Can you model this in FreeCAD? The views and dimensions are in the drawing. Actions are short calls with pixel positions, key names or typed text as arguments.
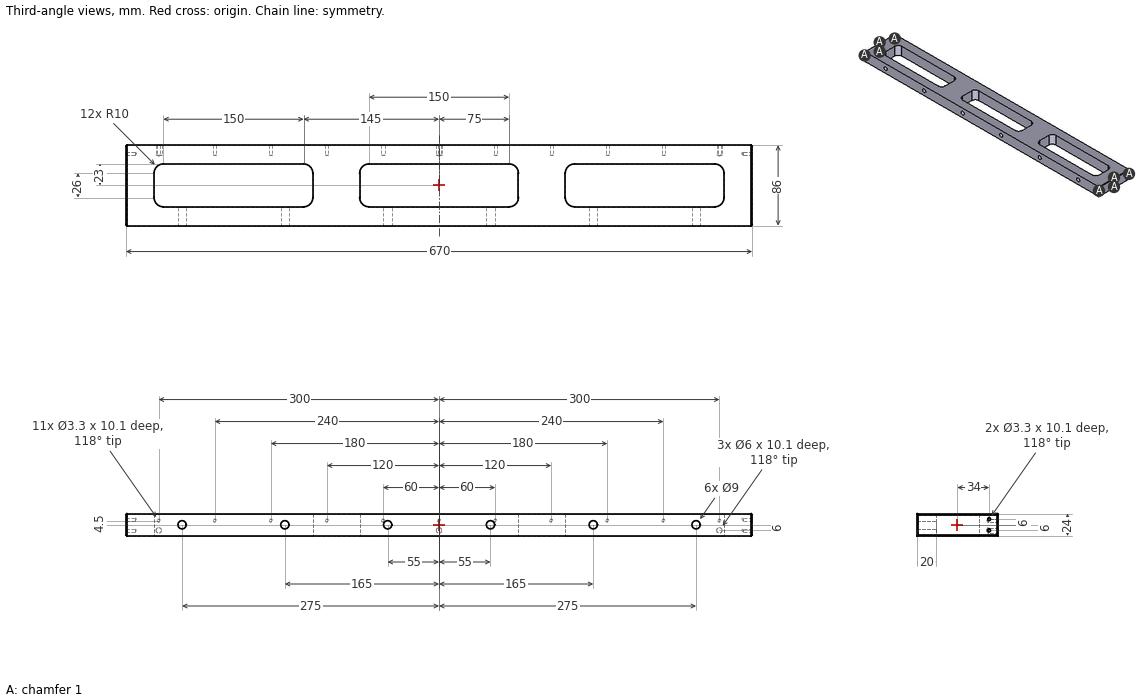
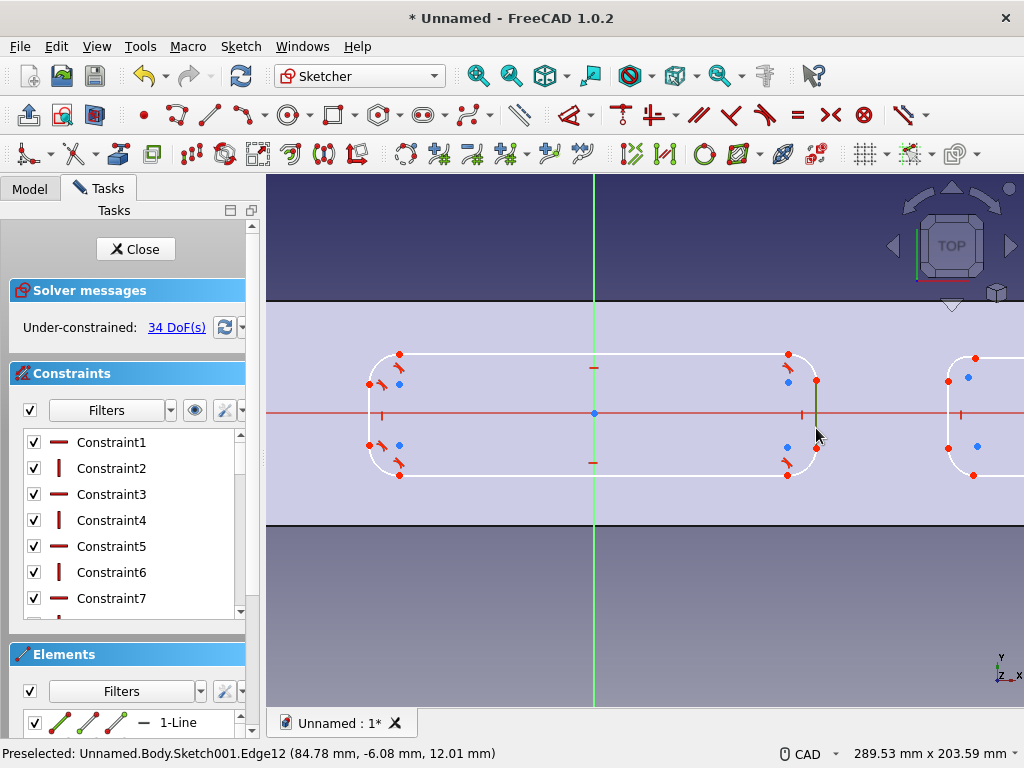
click(800, 473)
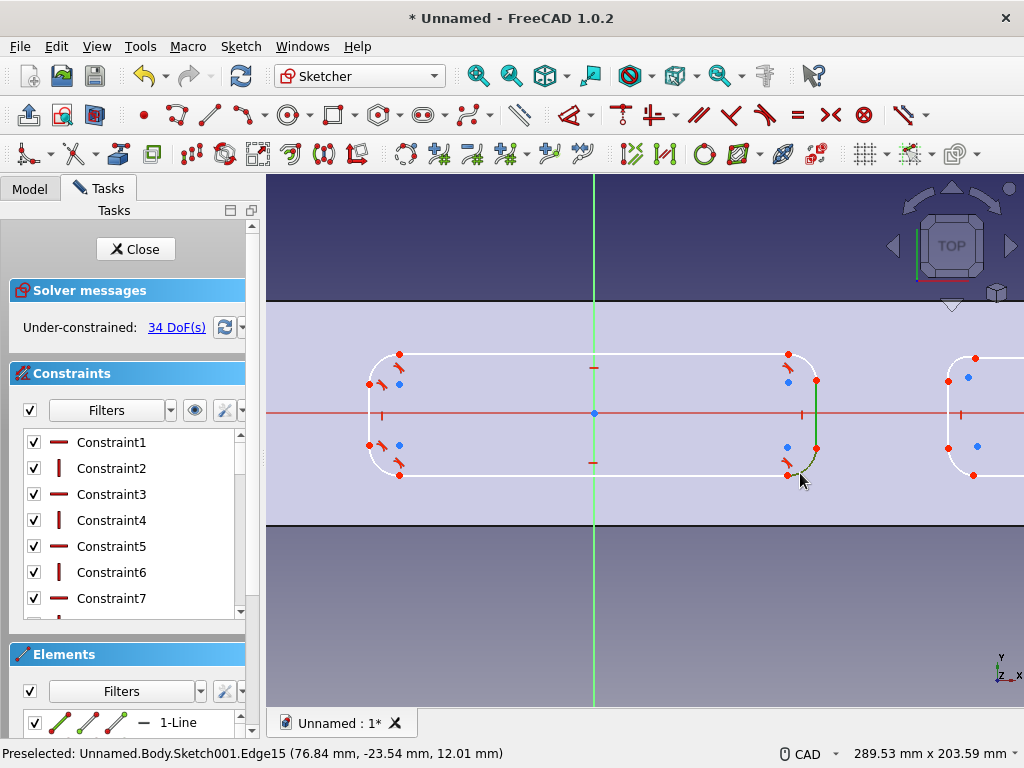
key(t)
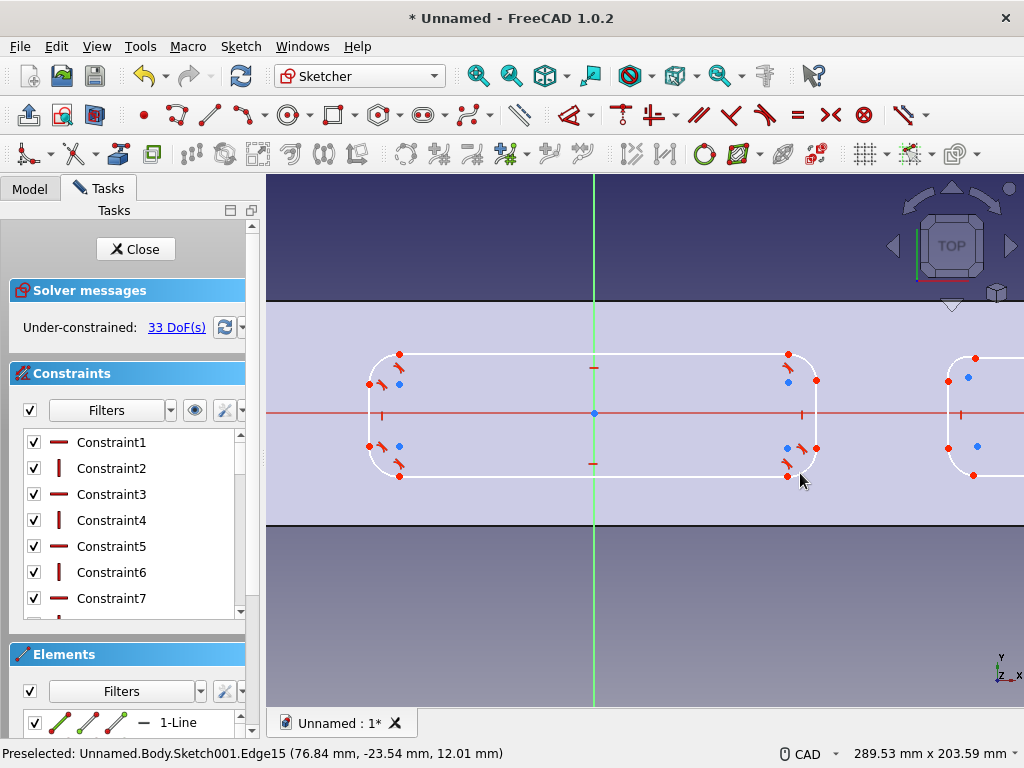
click(816, 428)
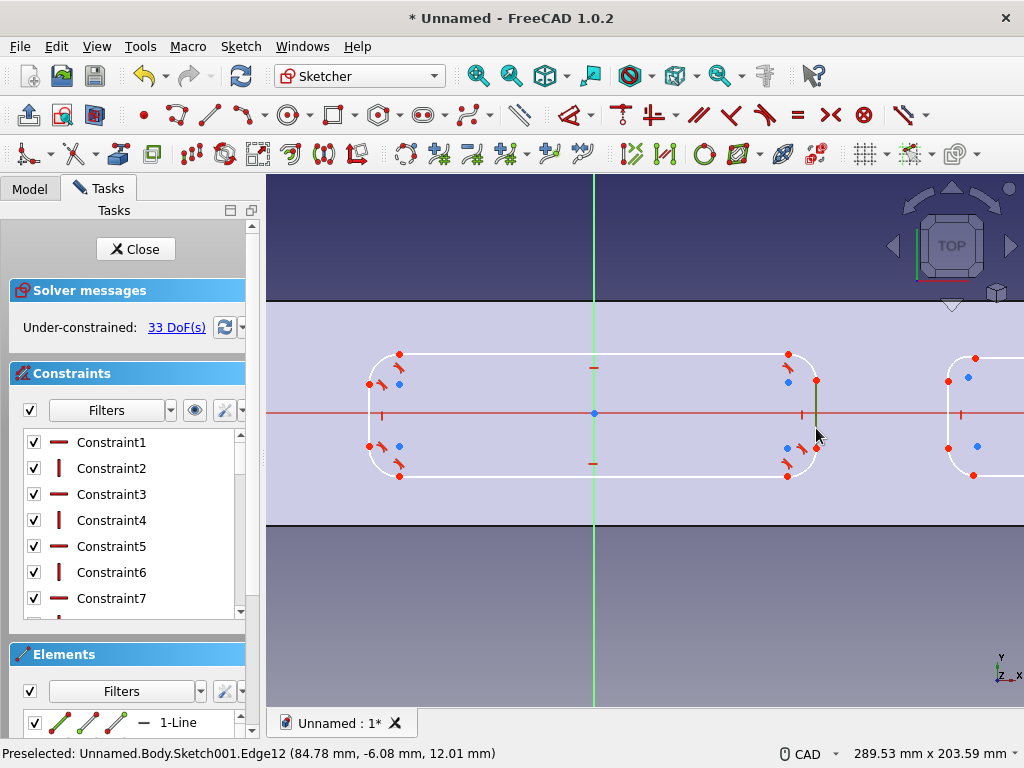
click(813, 369)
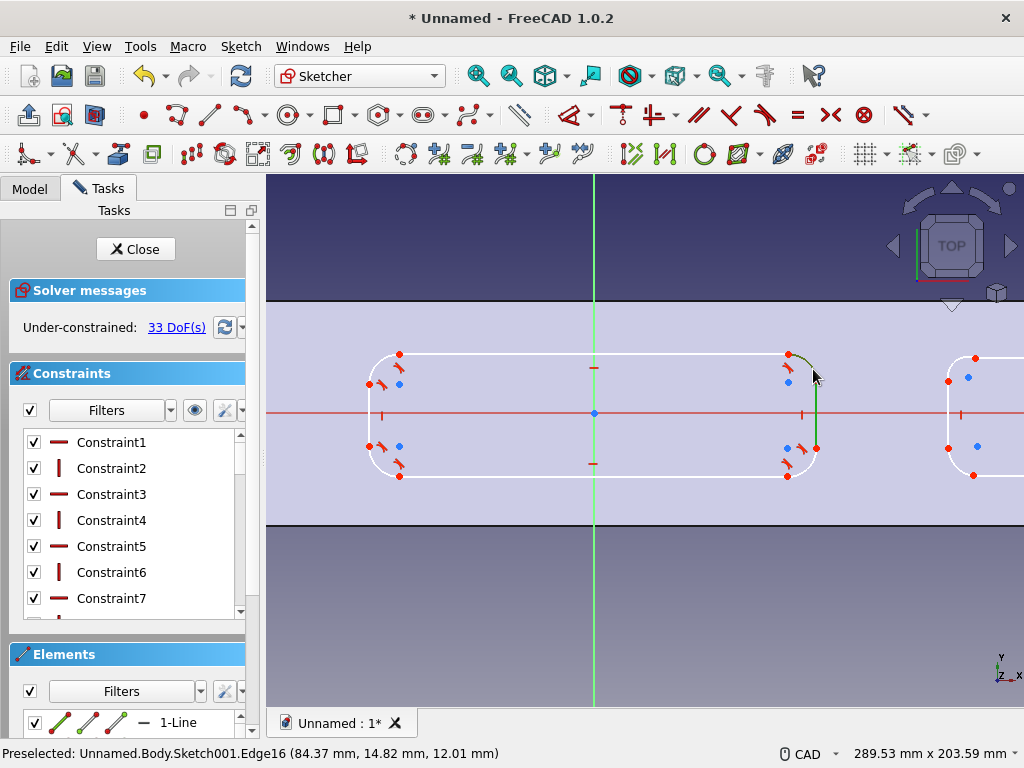
click(765, 116)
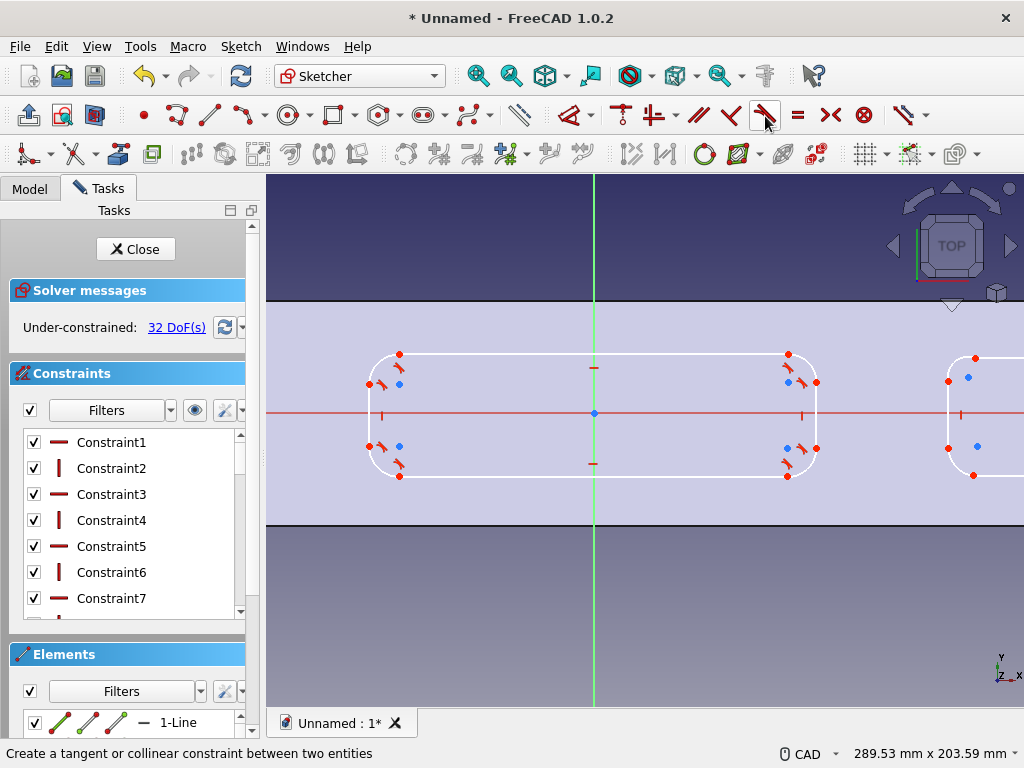
scroll(571, 449, down, 7)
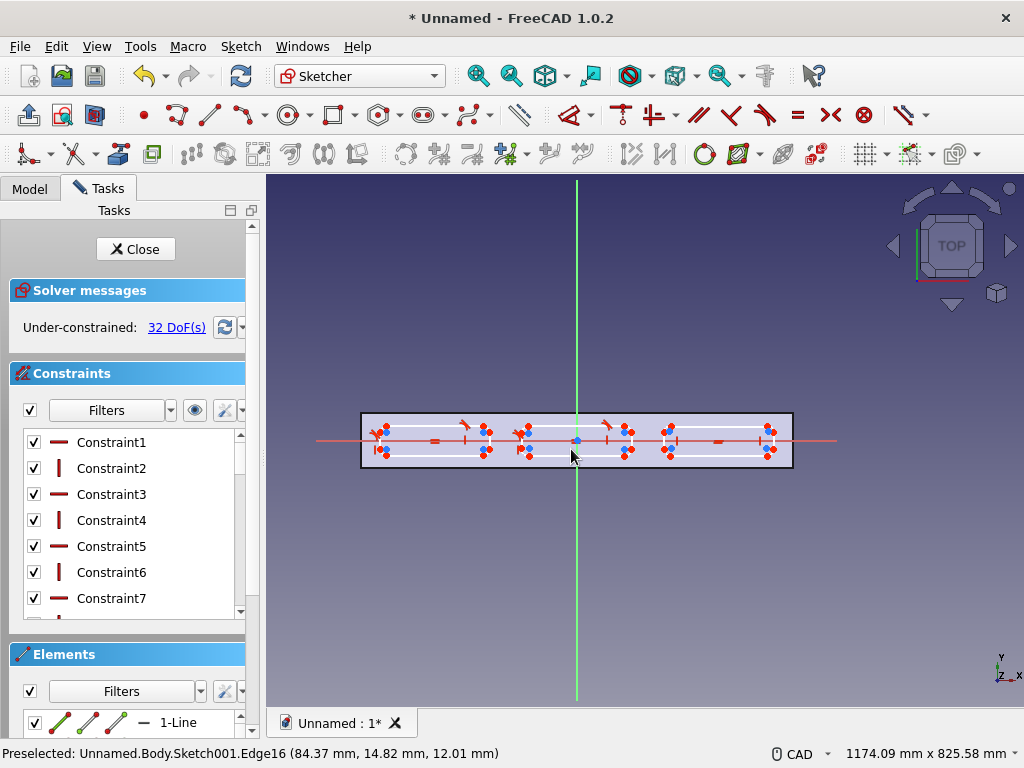
click(738, 427)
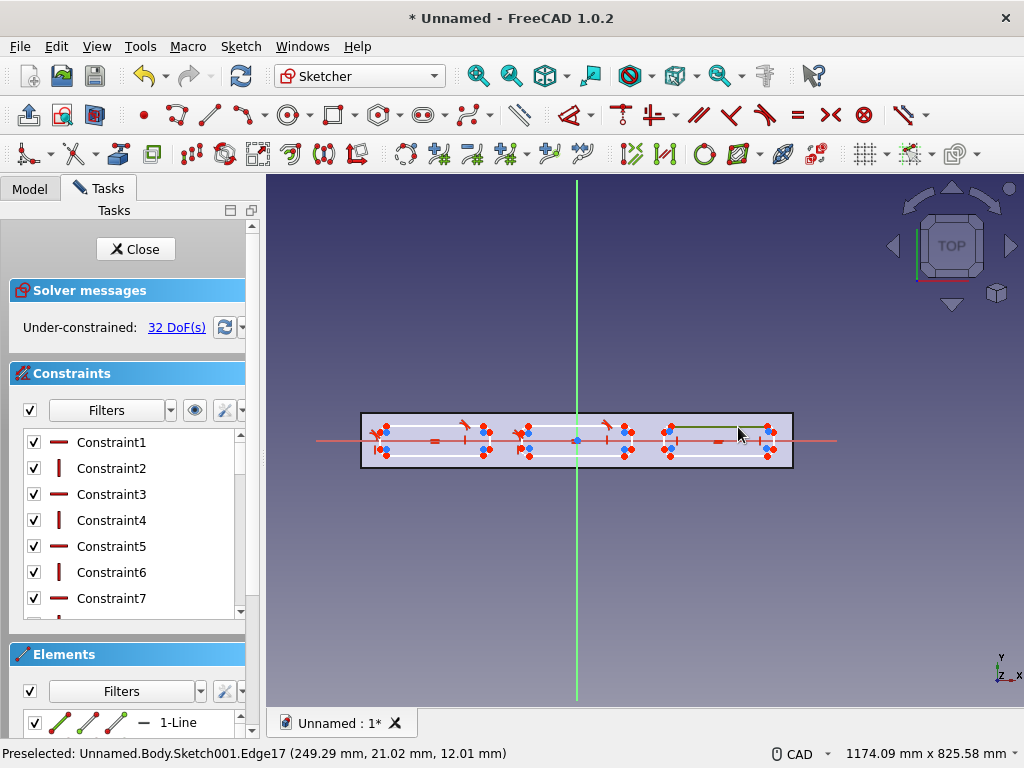
scroll(666, 428, up, 6)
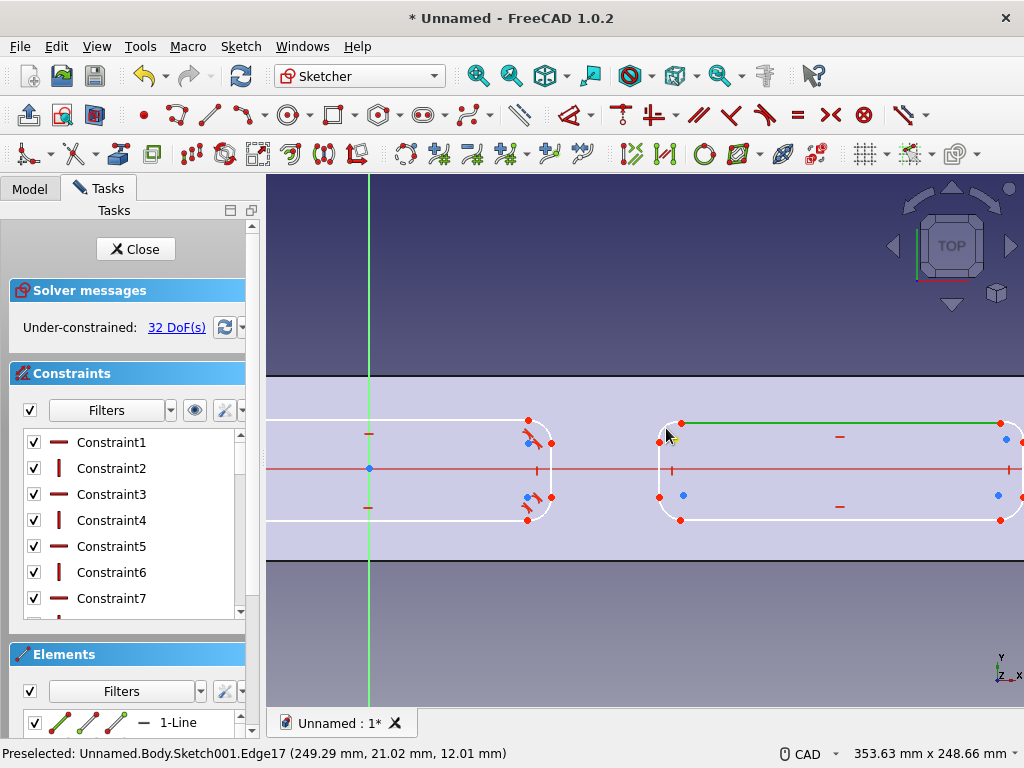
click(665, 426)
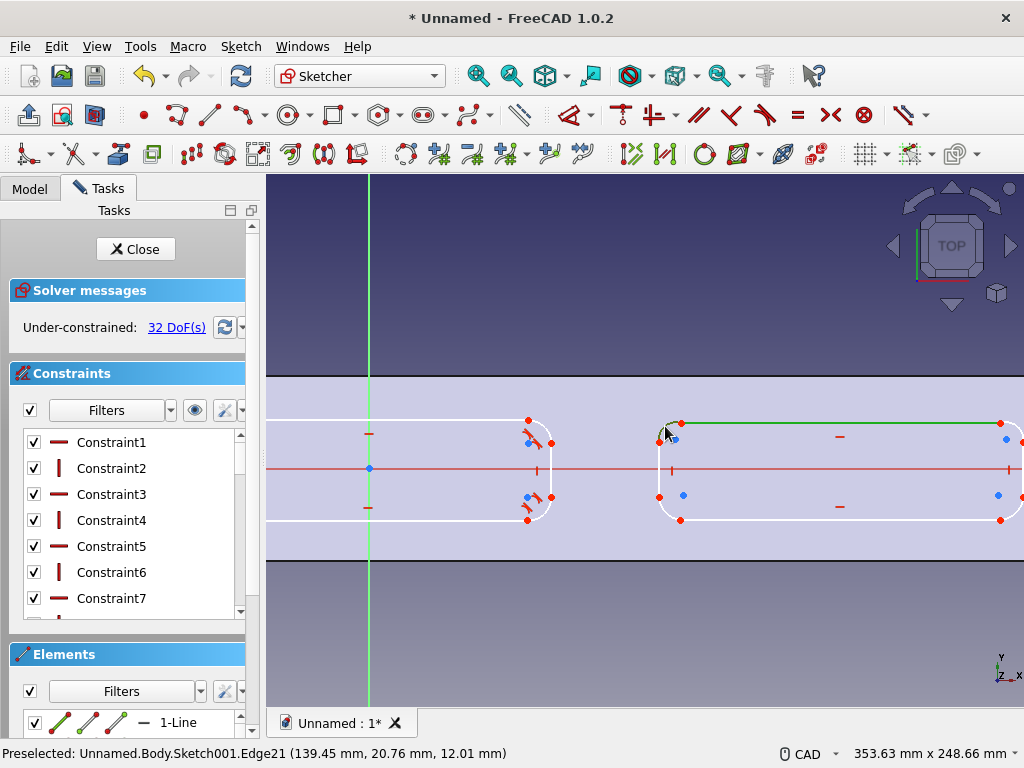
key(t)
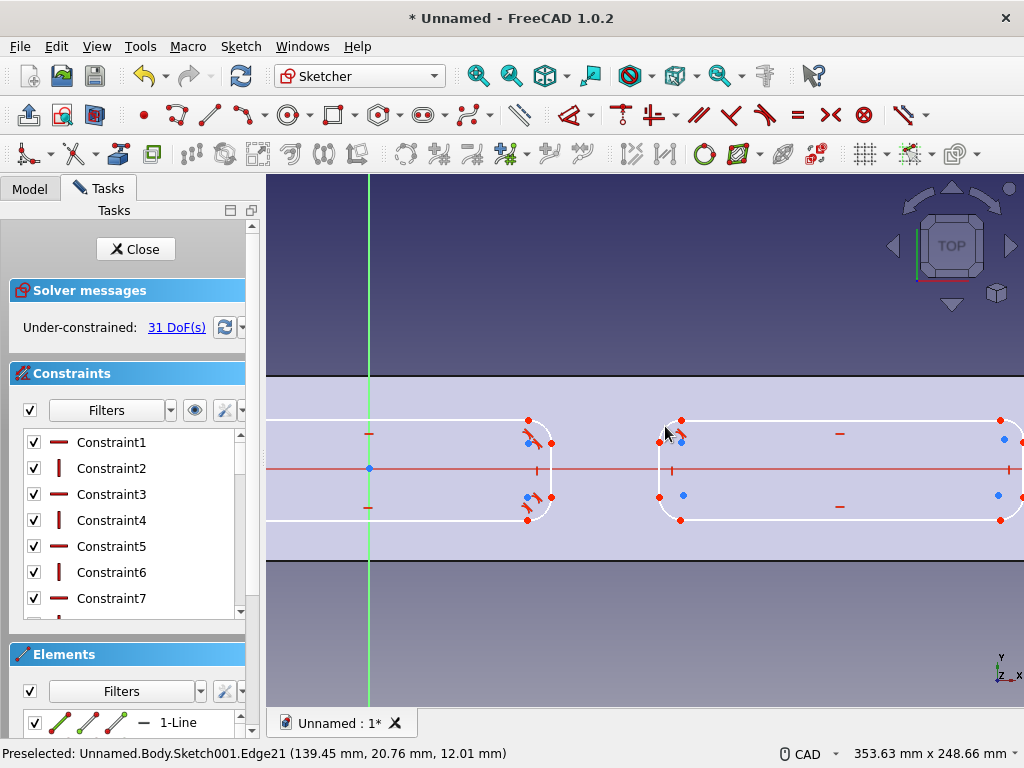
click(777, 421)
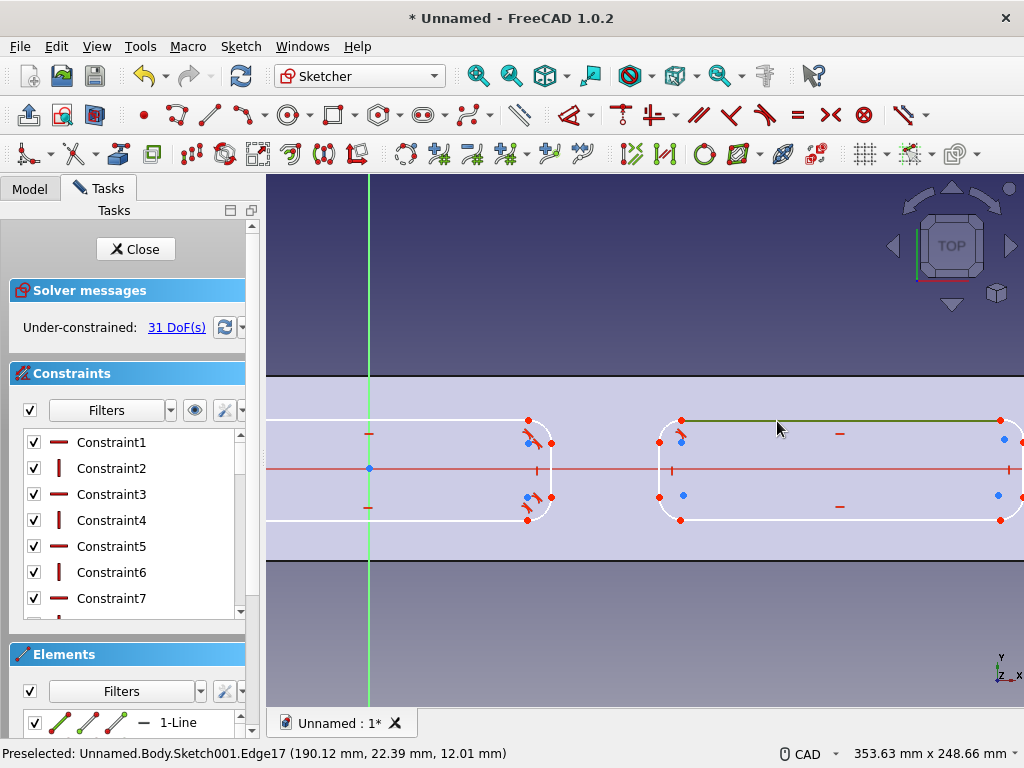
scroll(666, 428, down, 6)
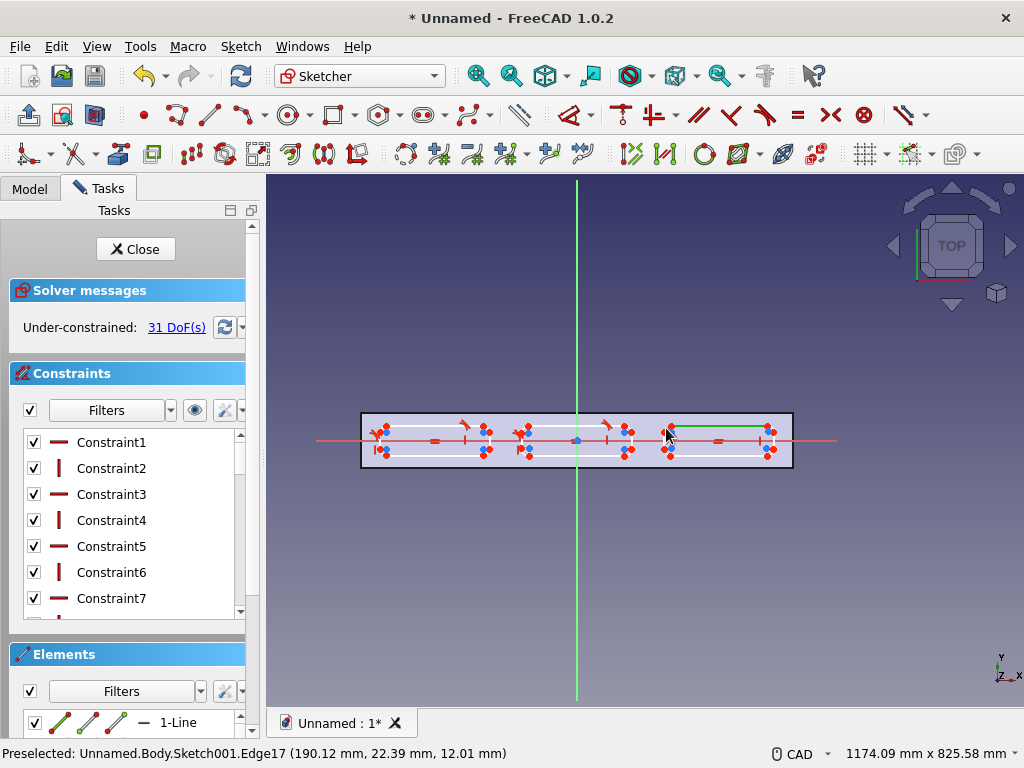
scroll(773, 429, up, 8)